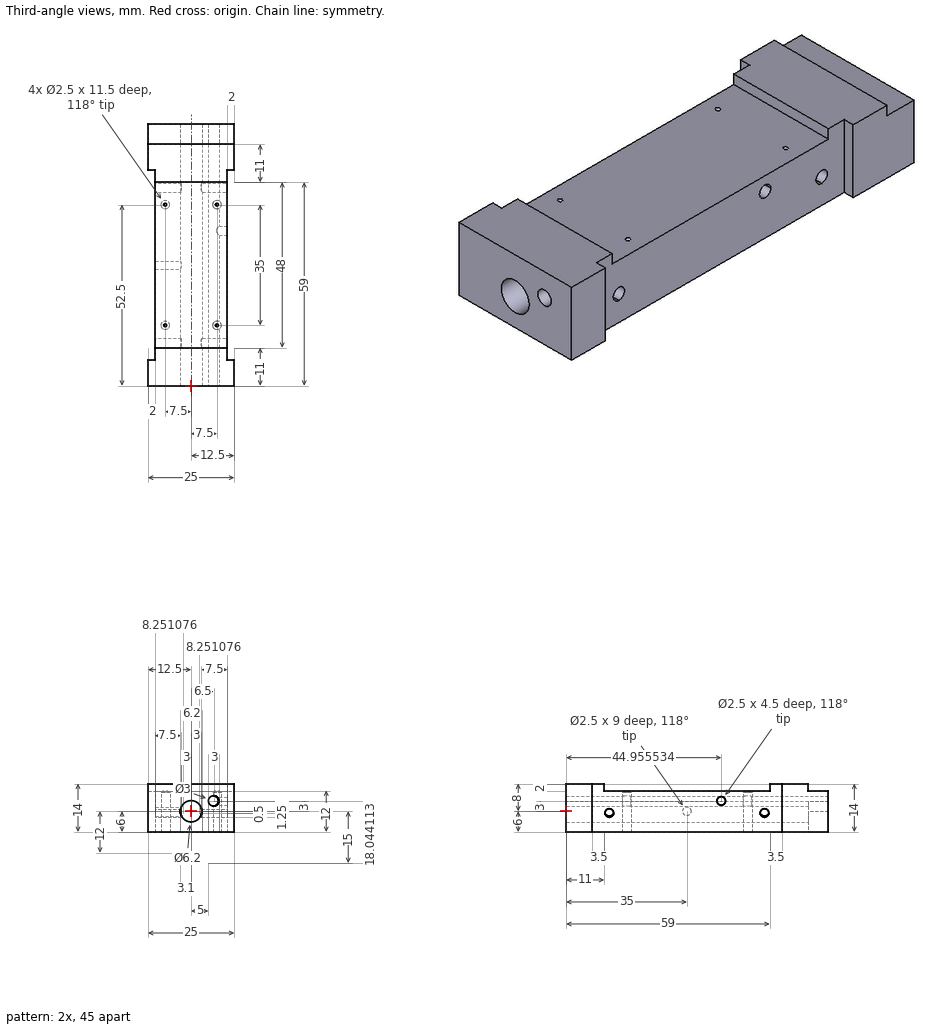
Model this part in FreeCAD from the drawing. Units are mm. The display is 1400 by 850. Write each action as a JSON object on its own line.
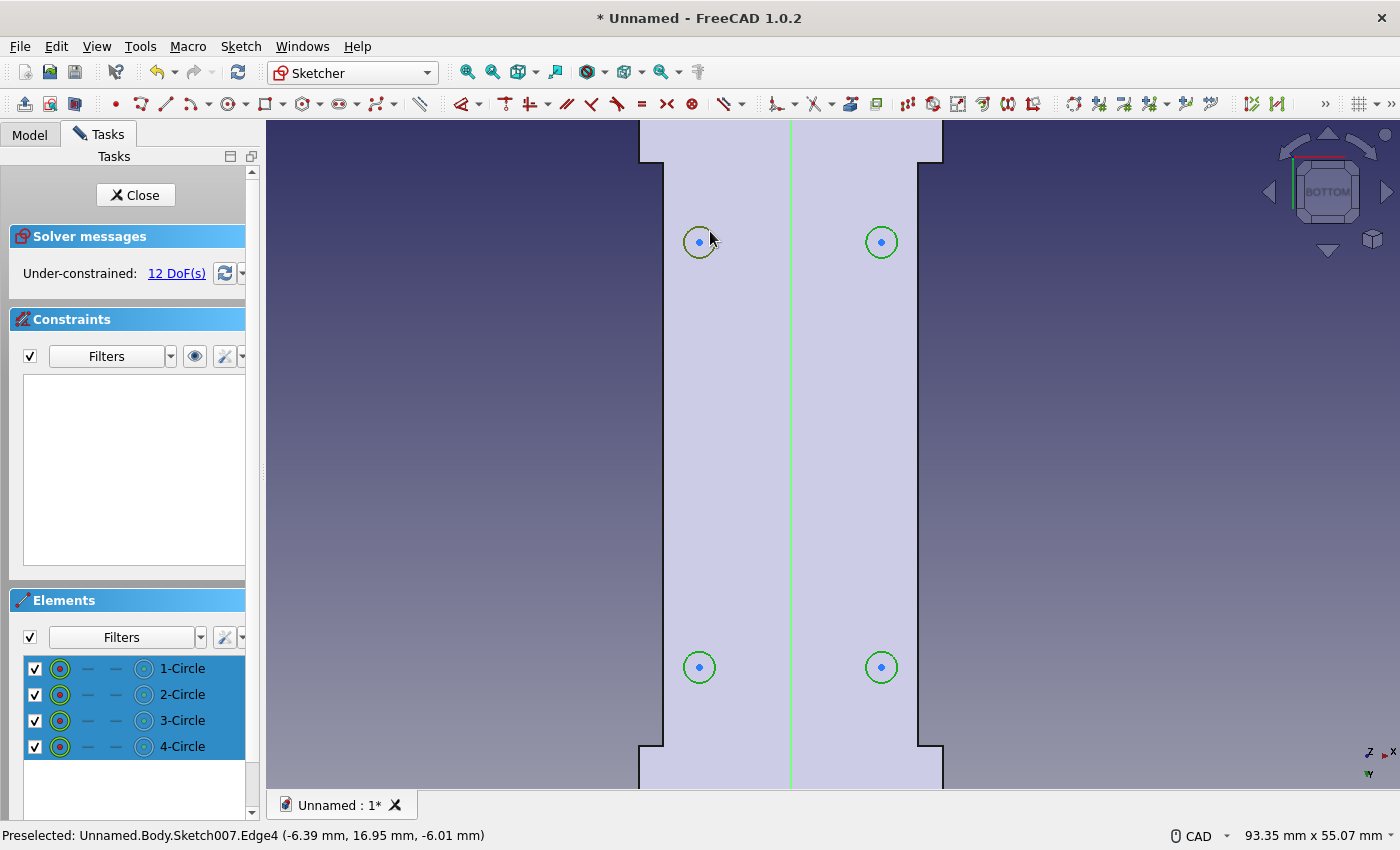
{"action": "left_click", "coordinate": [642, 104]}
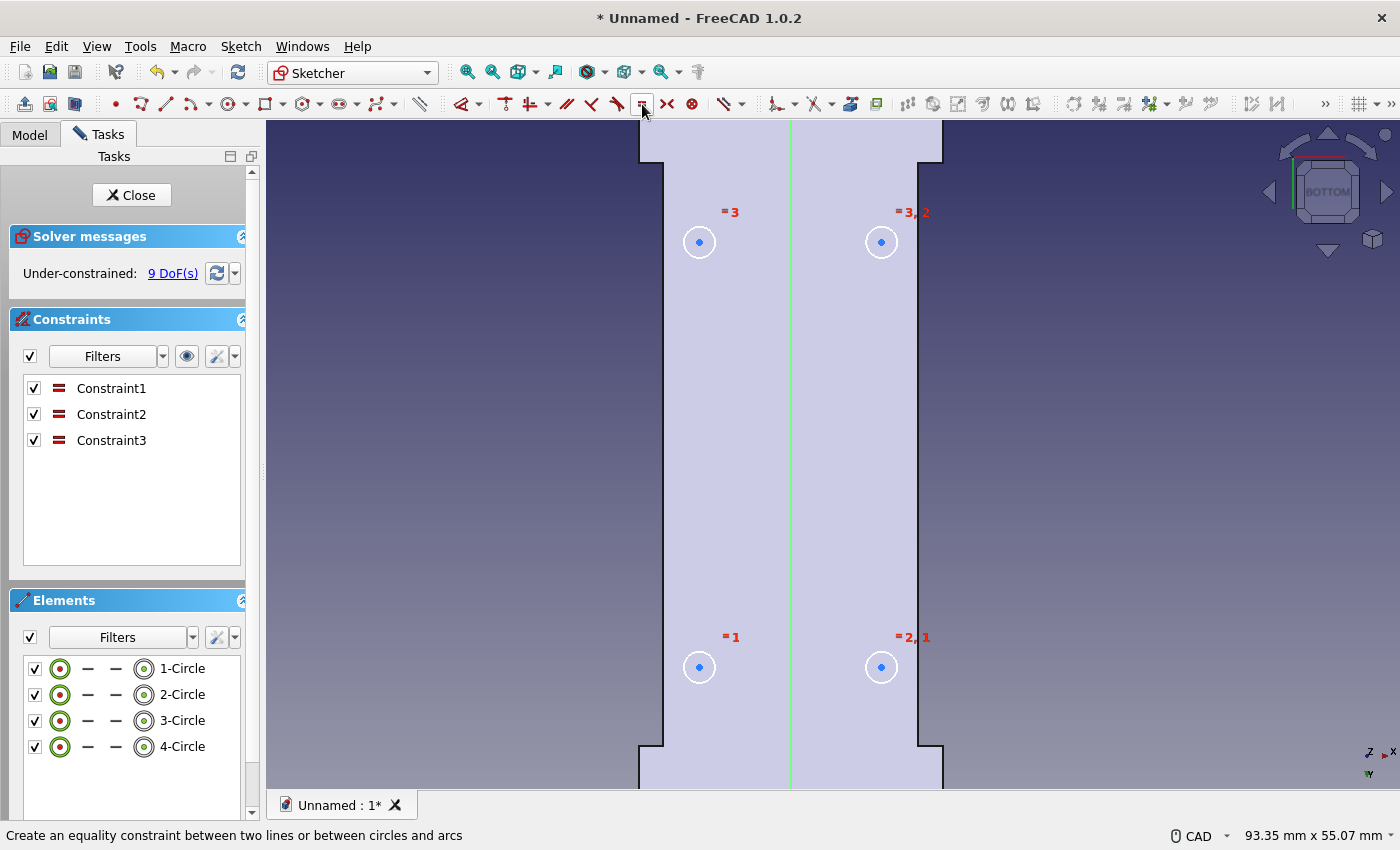
{"action": "left_click", "coordinate": [699, 667]}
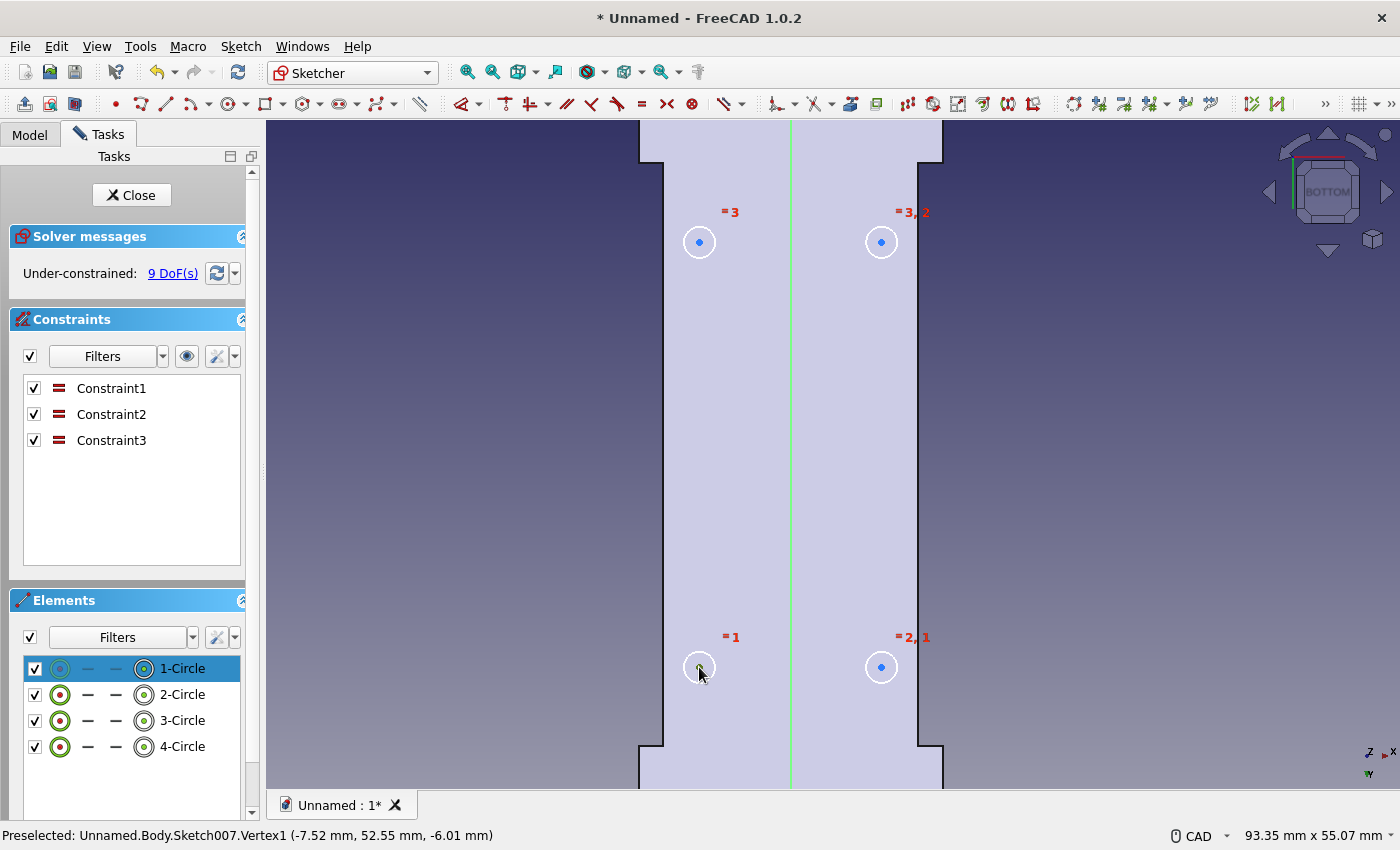
{"action": "left_click", "coordinate": [882, 667]}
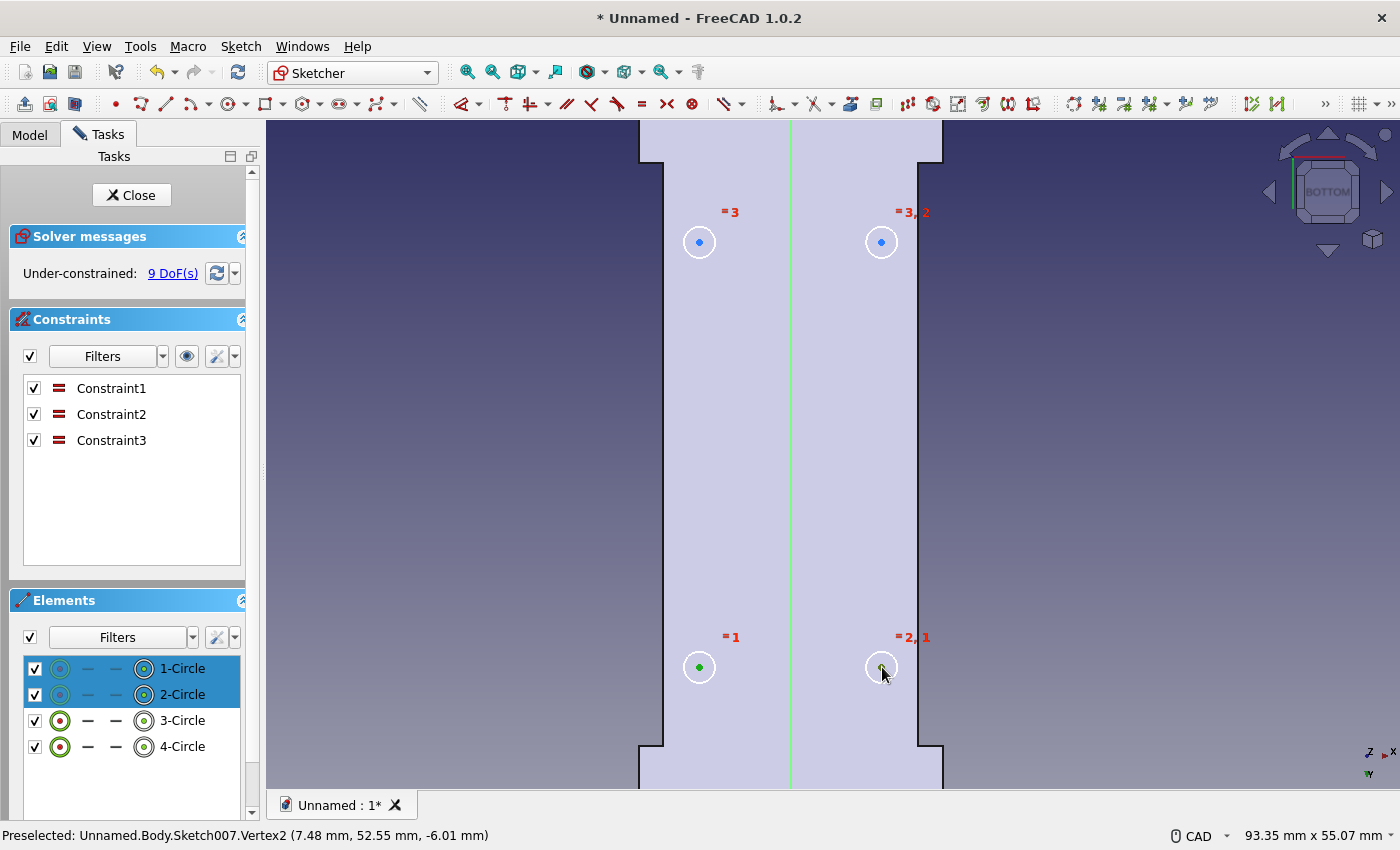
{"action": "key", "text": "h"}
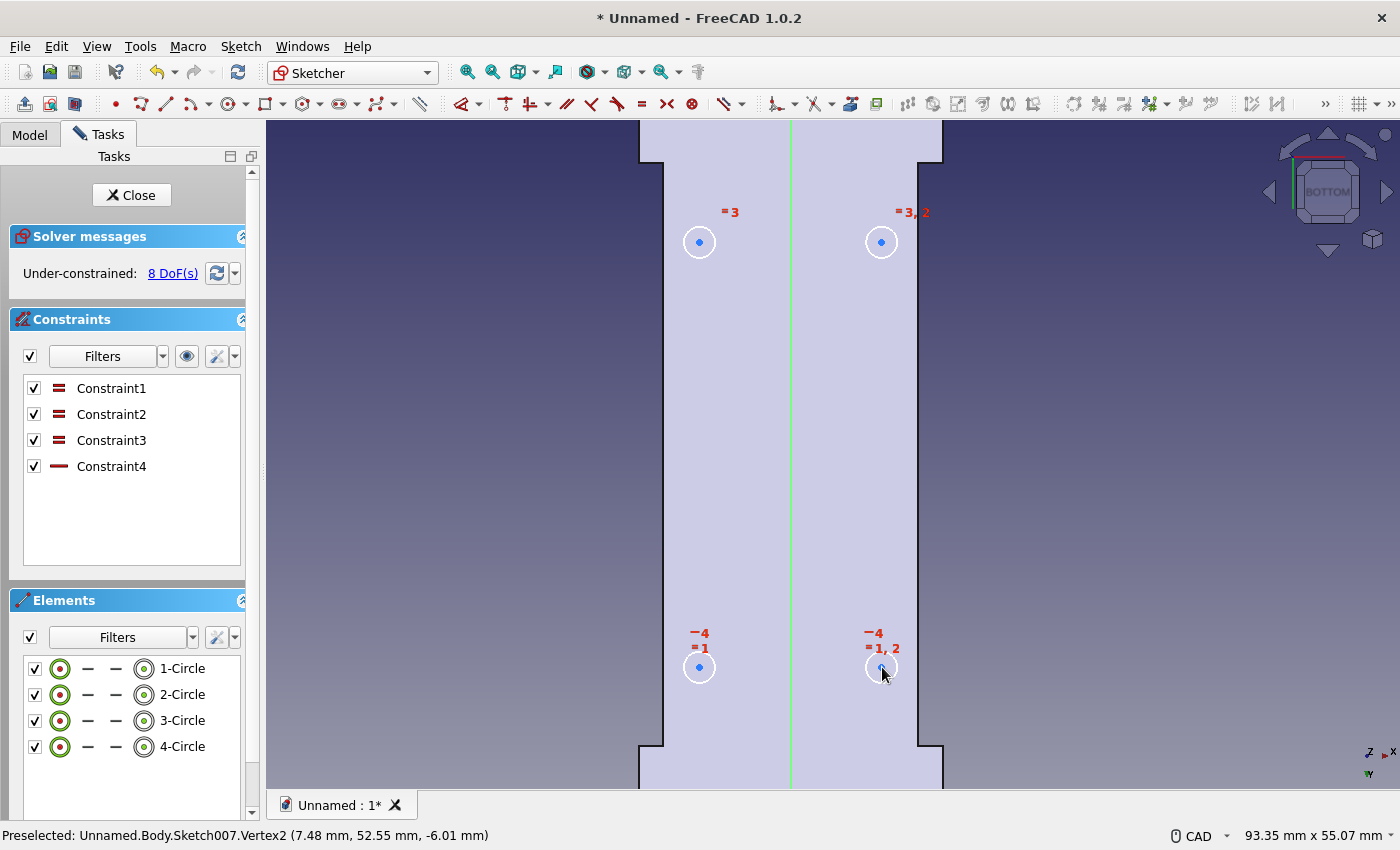
{"action": "left_click", "coordinate": [882, 667]}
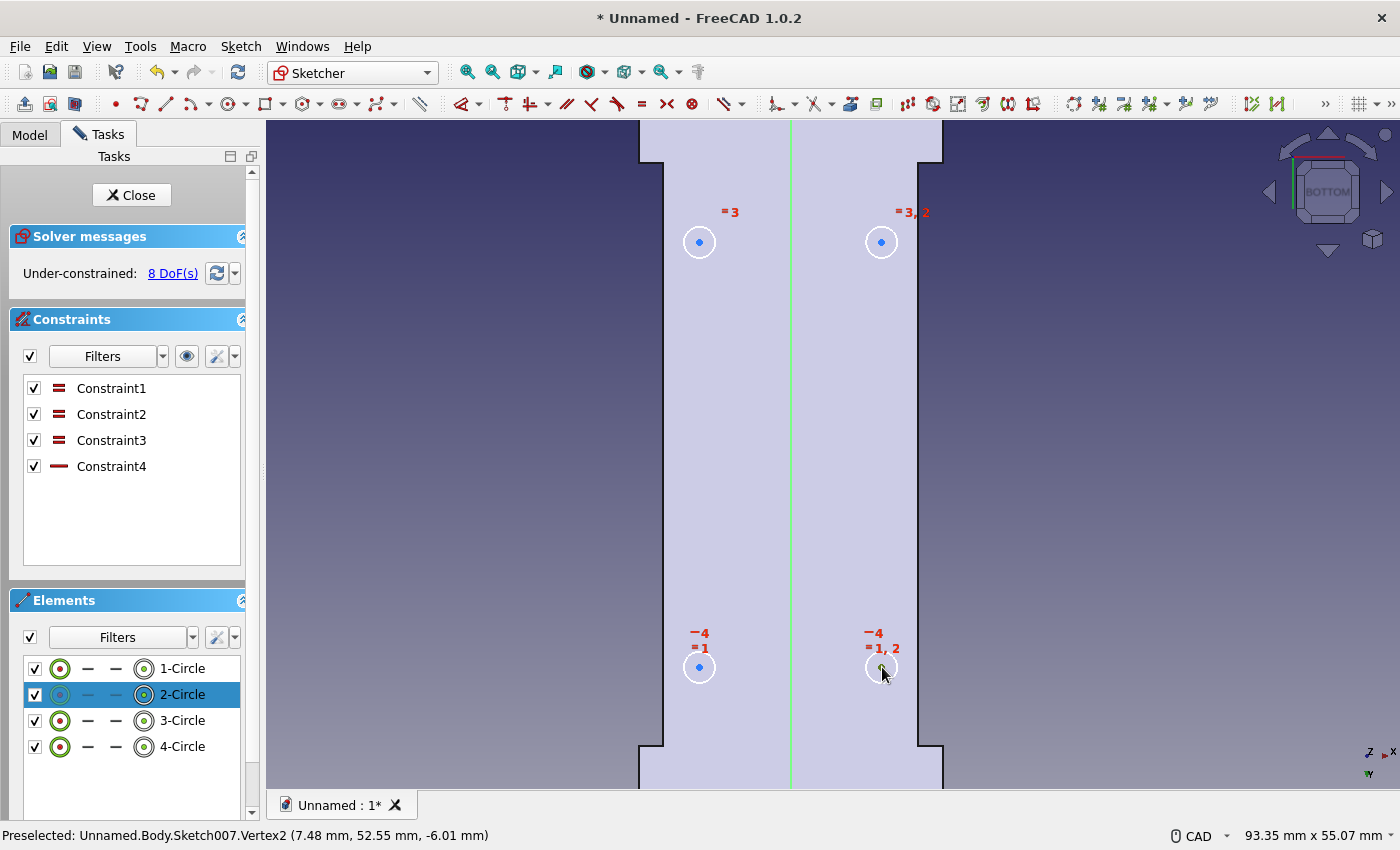
{"action": "left_click", "coordinate": [882, 242]}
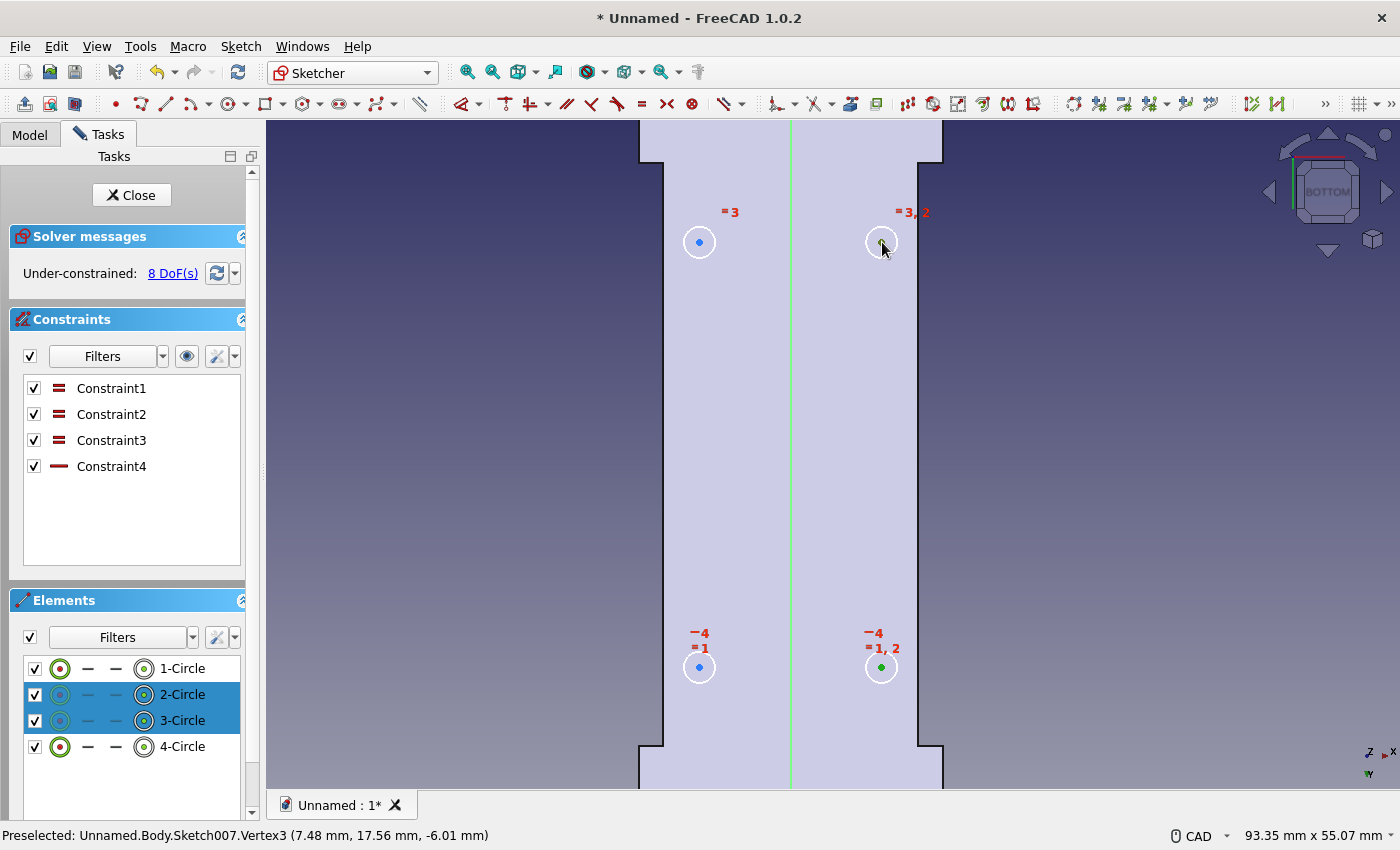
{"action": "left_click", "coordinate": [548, 104]}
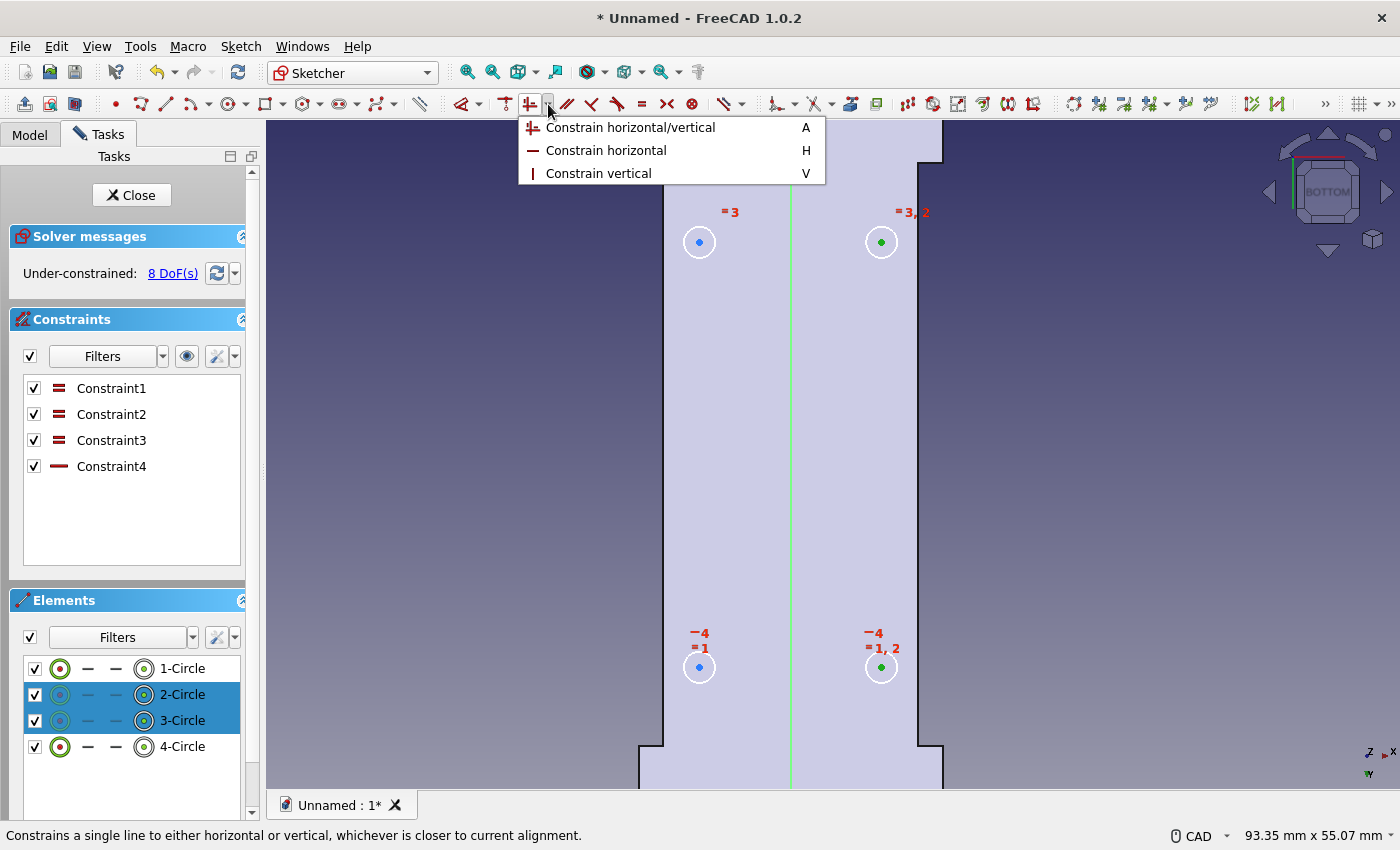
{"action": "left_click", "coordinate": [672, 174]}